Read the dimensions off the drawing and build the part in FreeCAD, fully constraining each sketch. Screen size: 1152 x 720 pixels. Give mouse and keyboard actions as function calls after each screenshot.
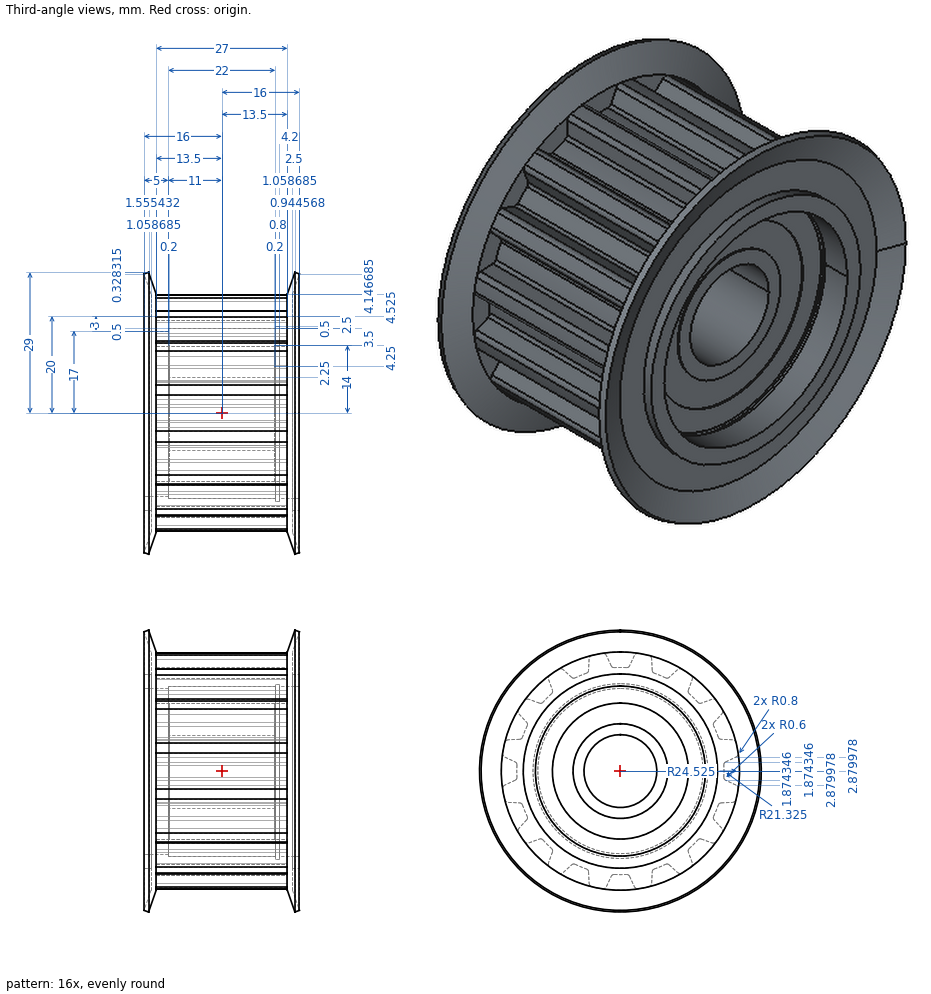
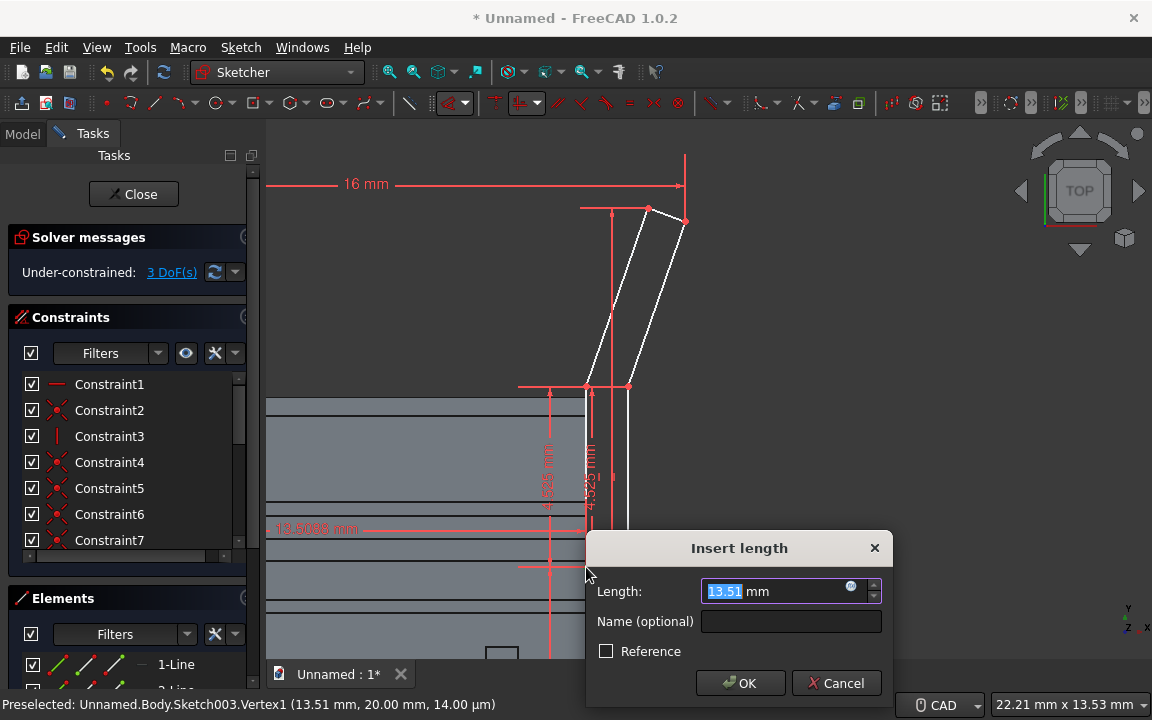
text(13.5)
key(Return)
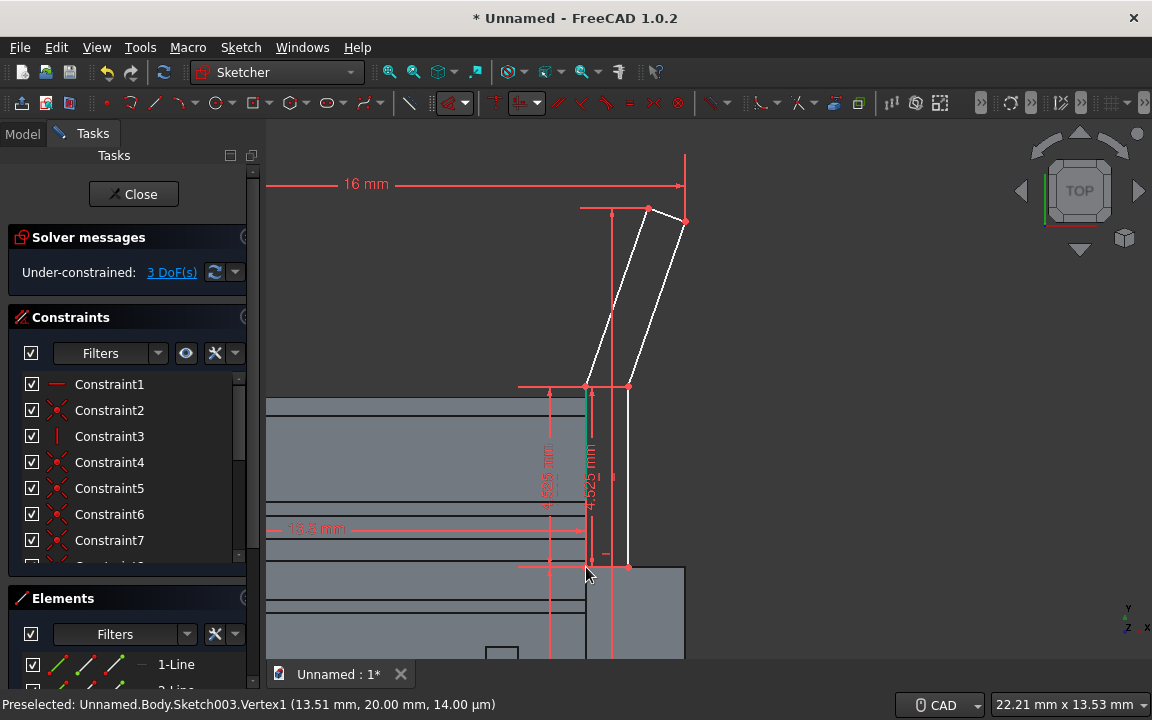
click(598, 567)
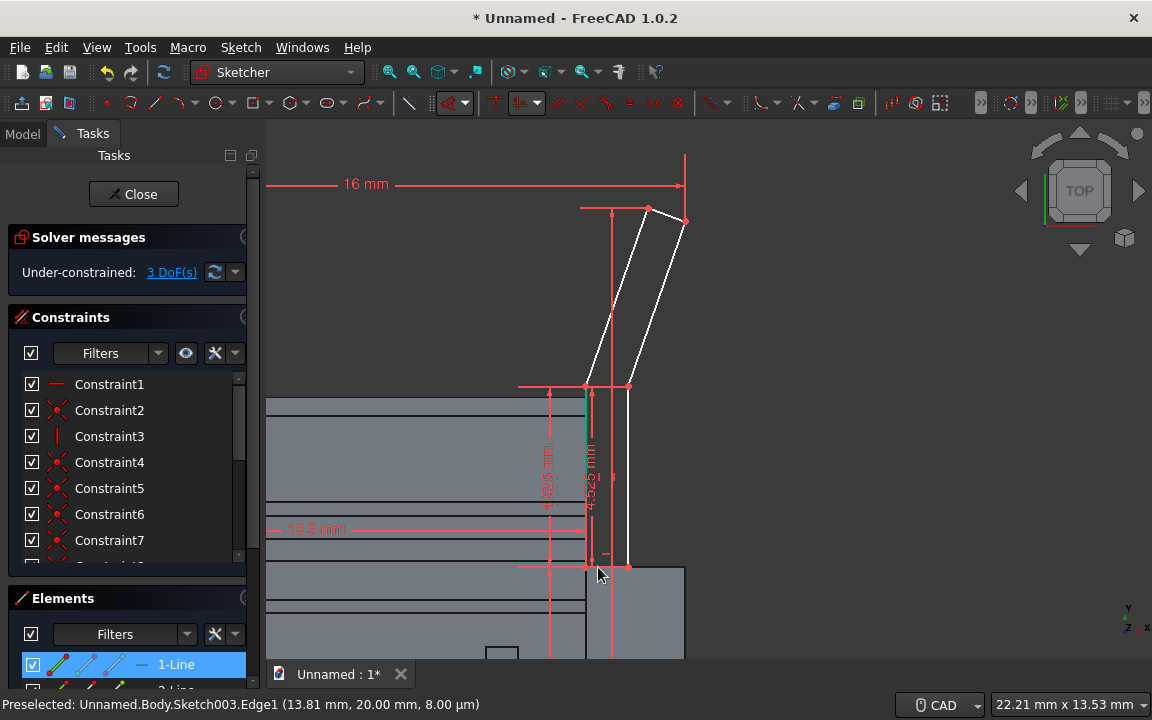
click(468, 104)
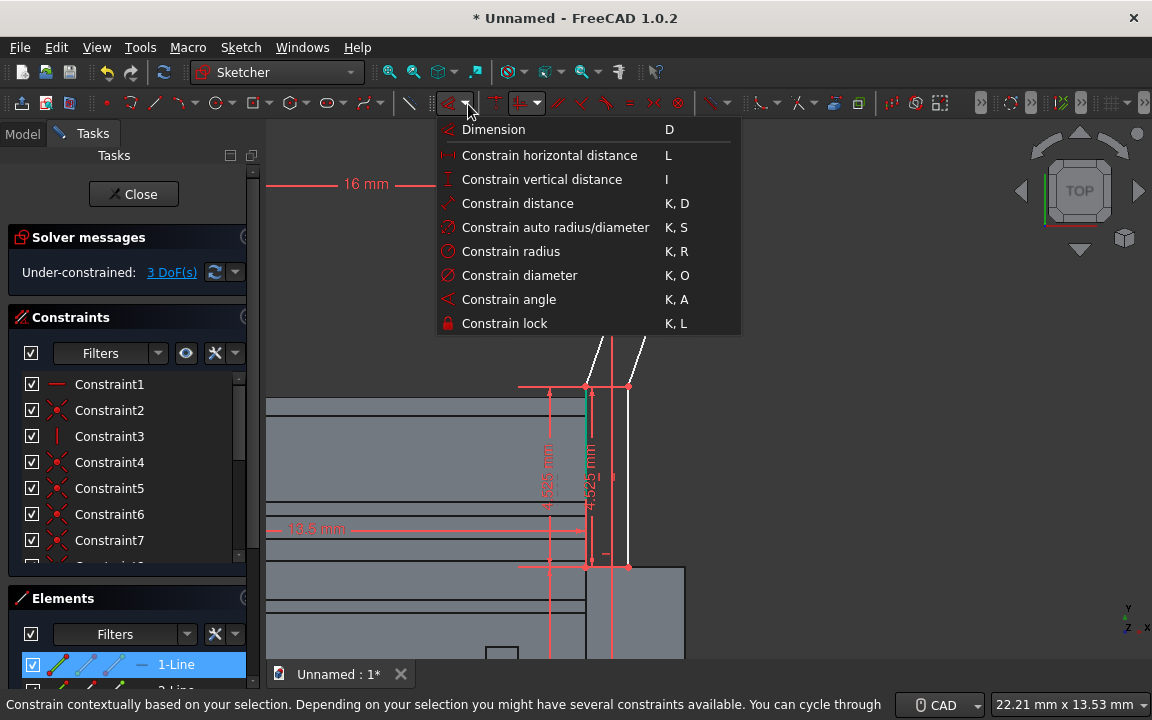
click(589, 155)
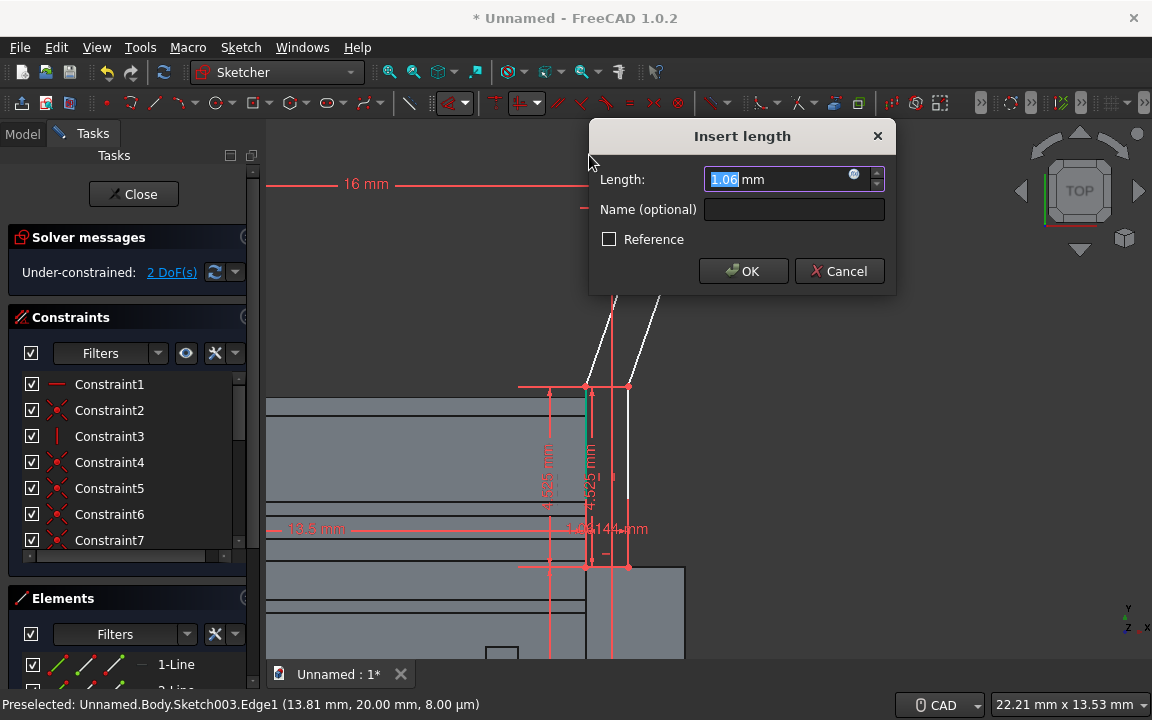
text(1.058685)
key(Return)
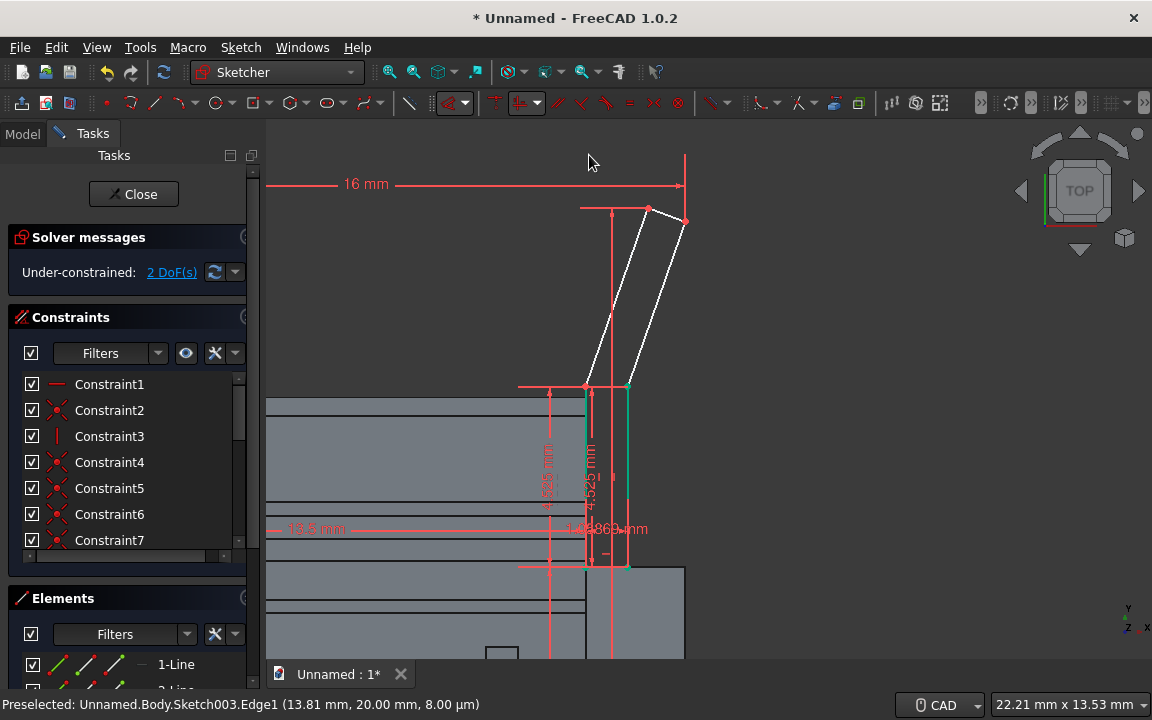
click(645, 337)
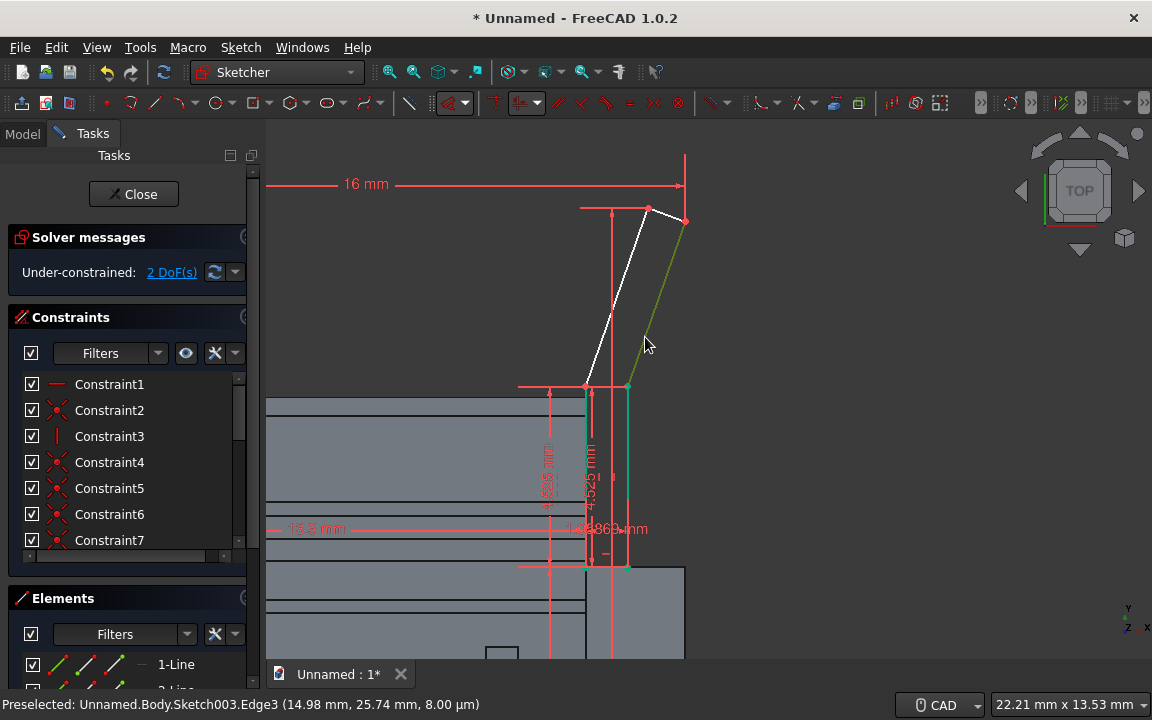
click(468, 104)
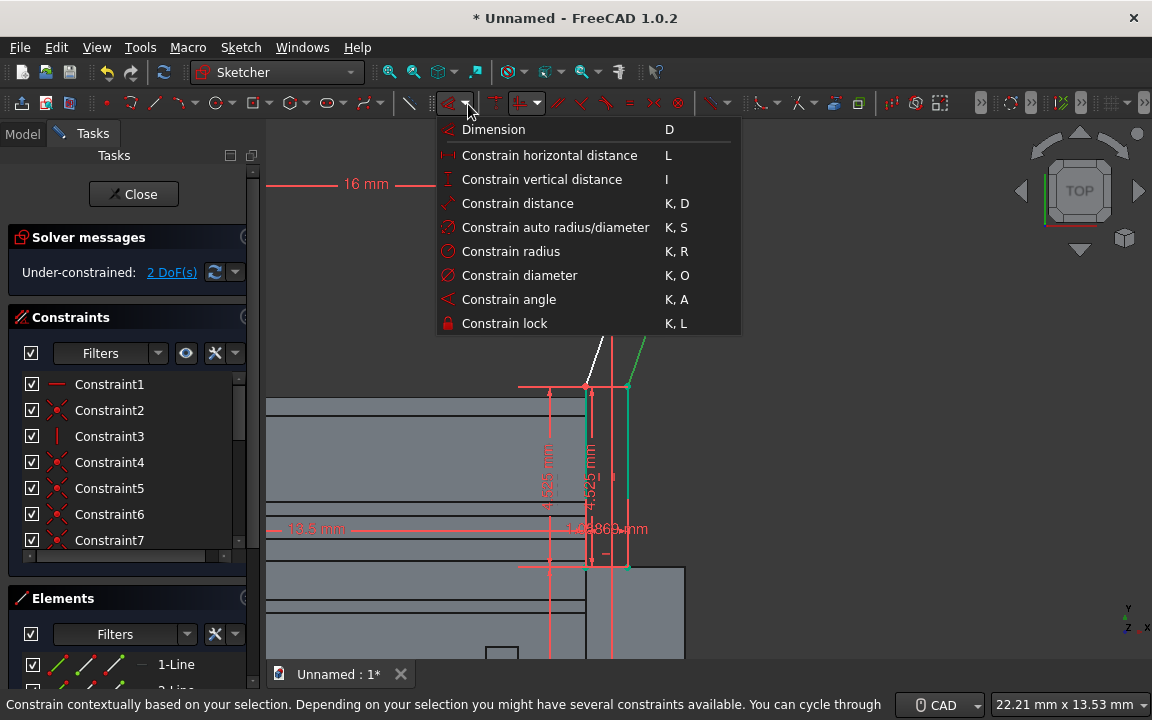
click(589, 179)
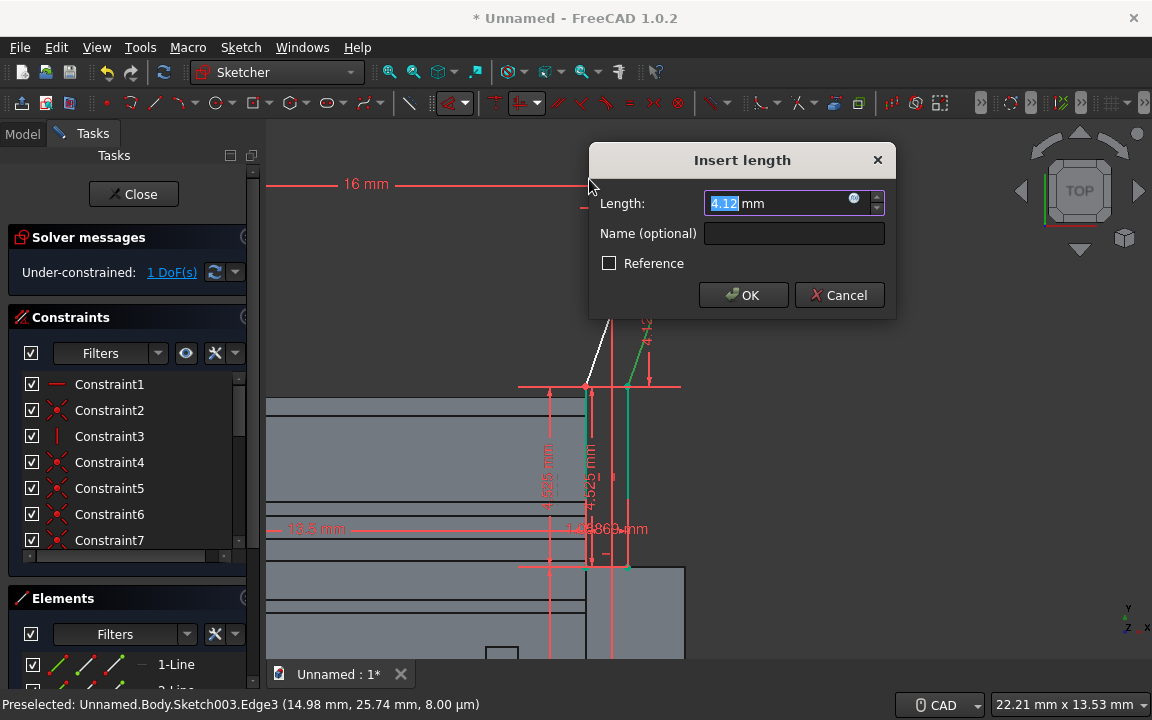
text(4.146685)
key(Return)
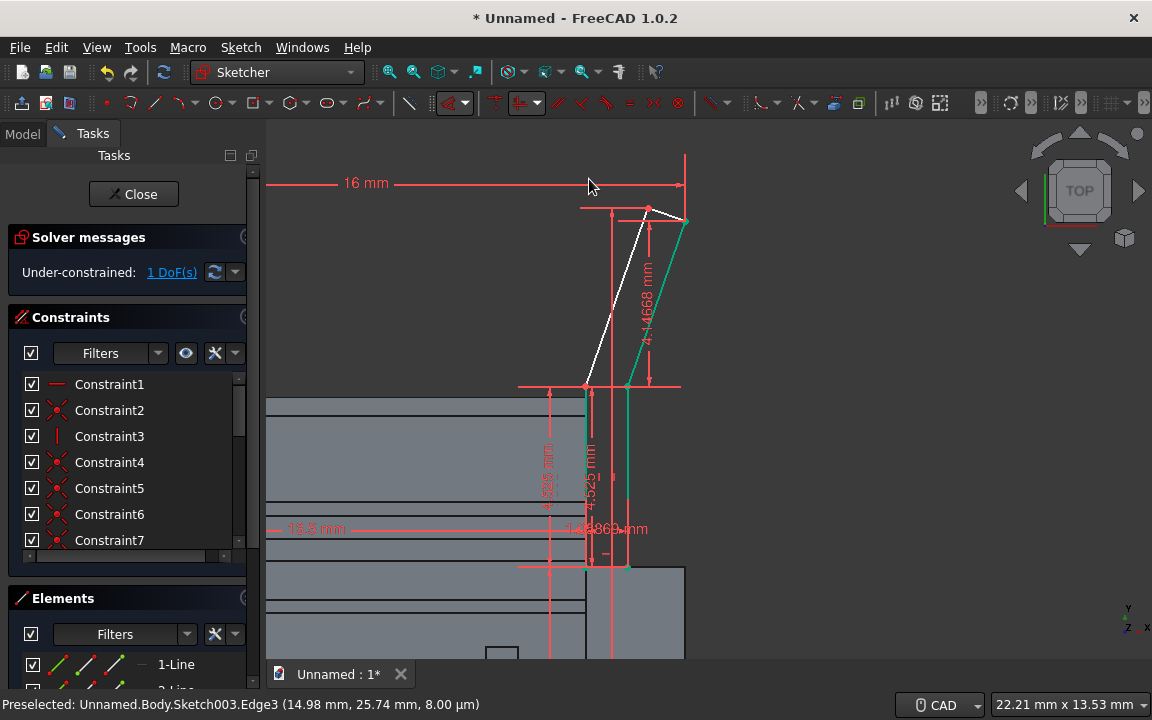
click(674, 217)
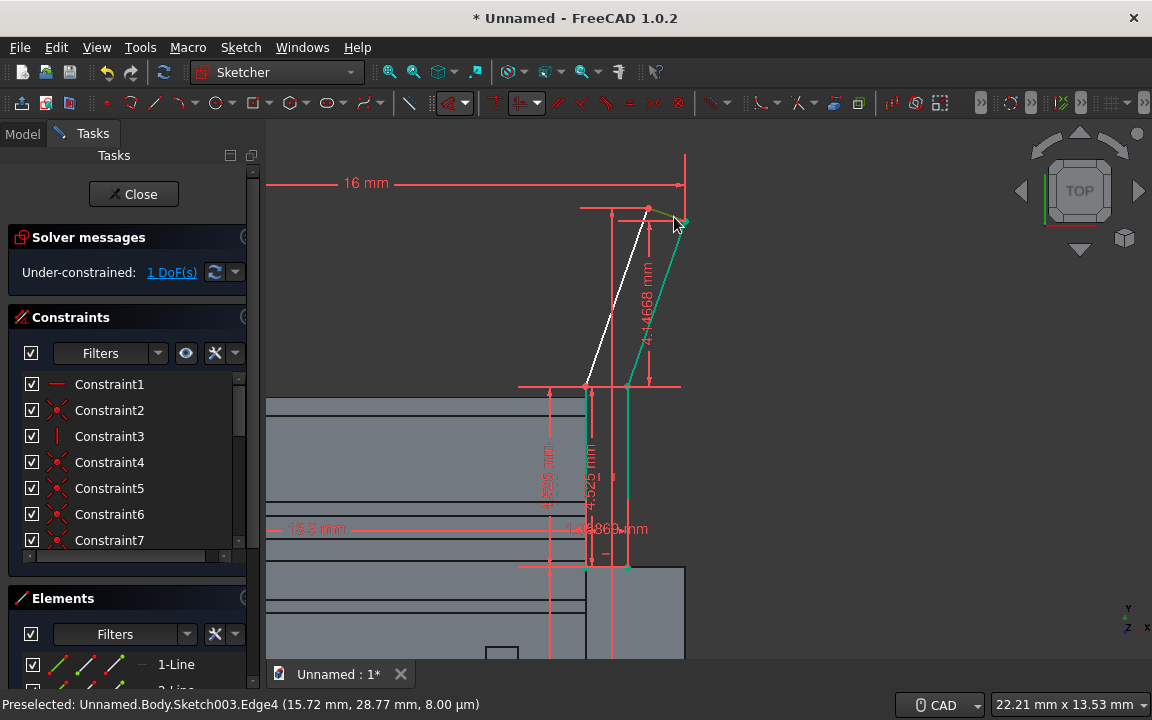
click(468, 104)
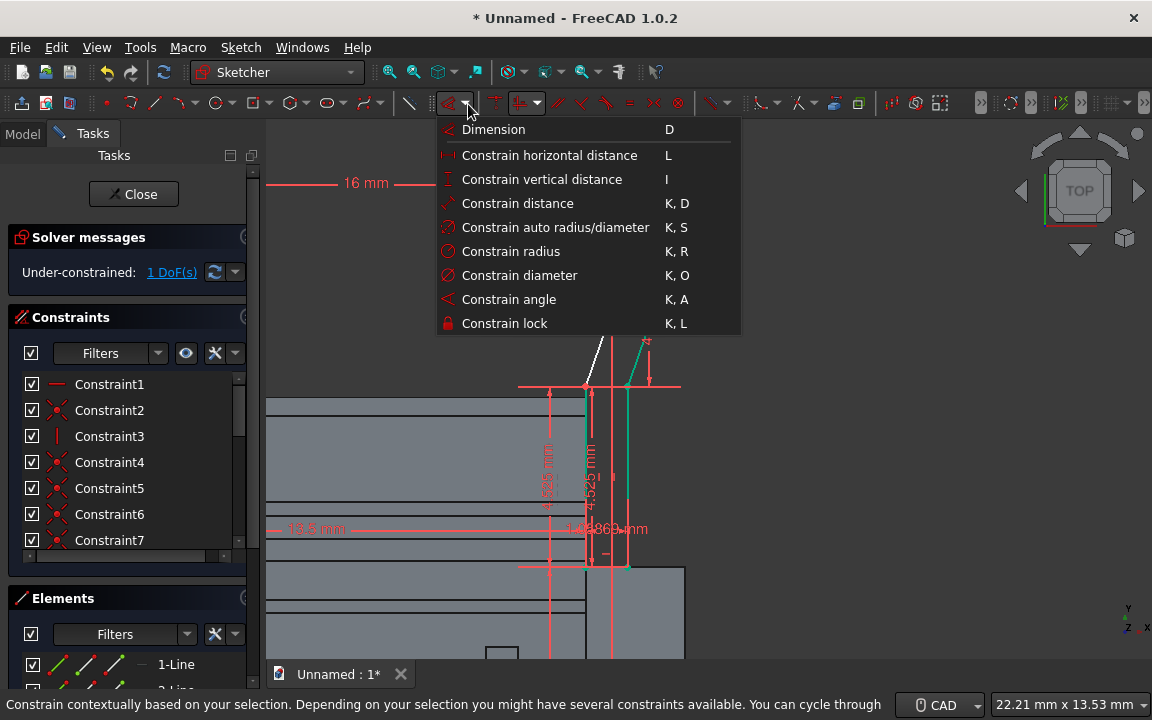
click(589, 155)